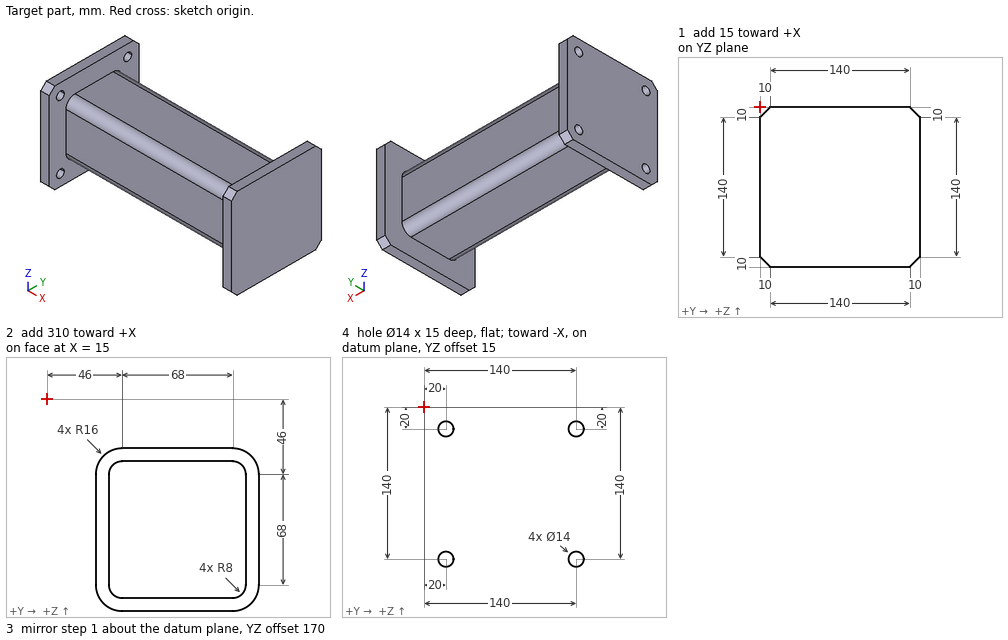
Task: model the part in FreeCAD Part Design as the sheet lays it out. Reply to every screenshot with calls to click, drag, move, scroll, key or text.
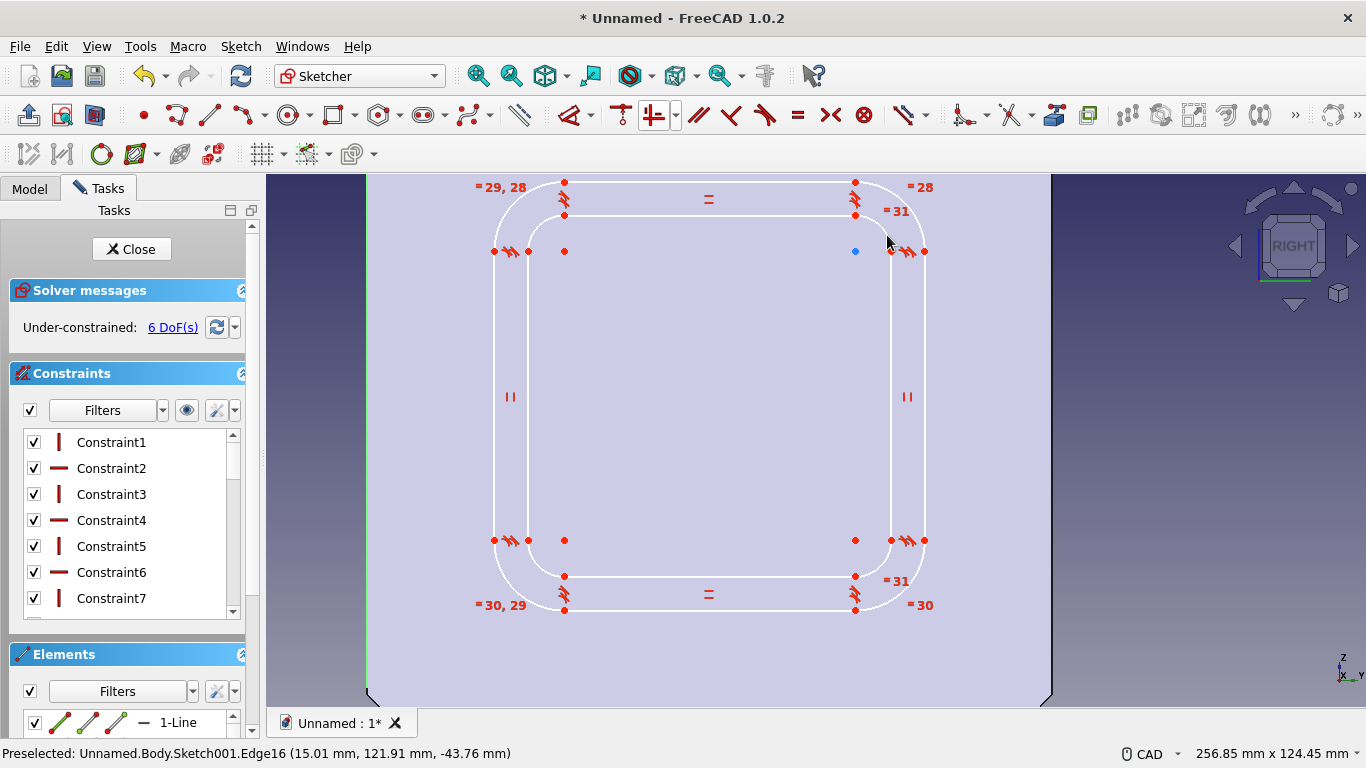
click(568, 116)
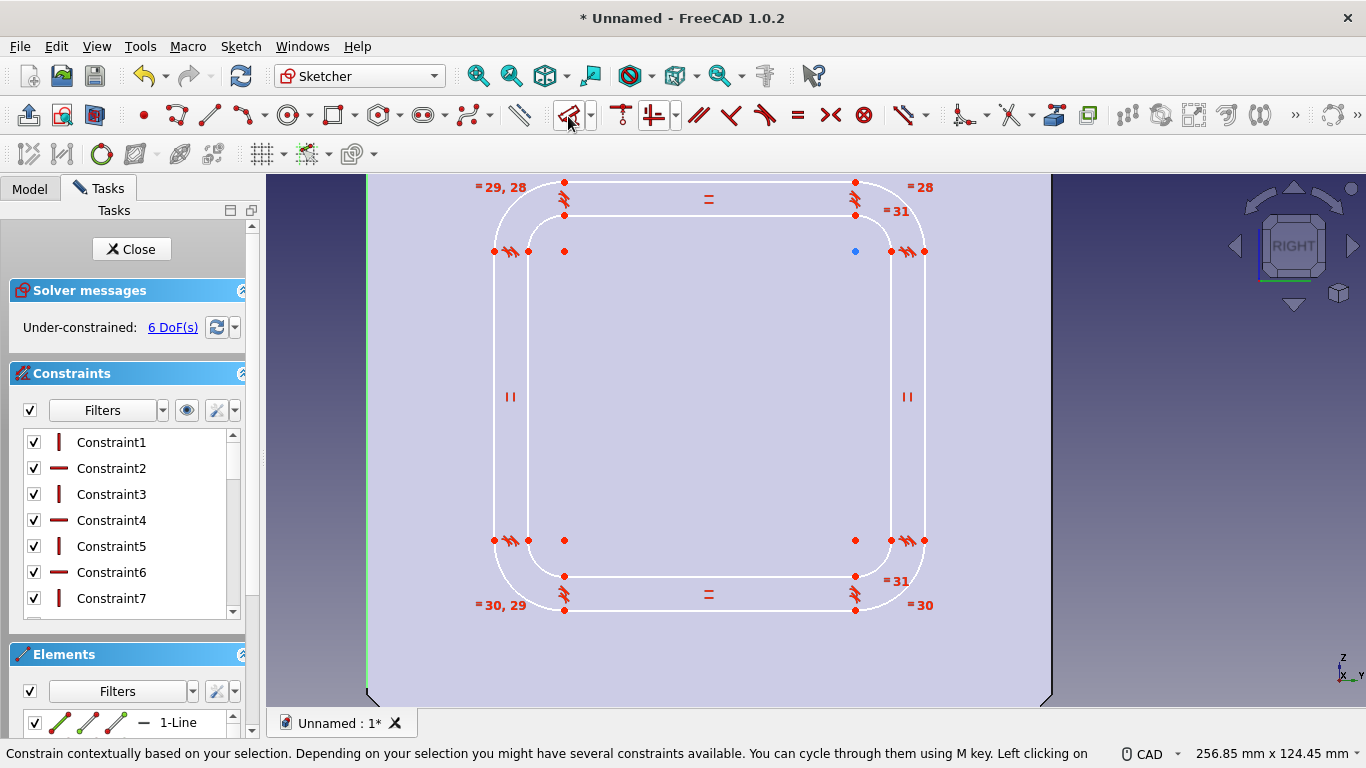
click(917, 220)
click(945, 205)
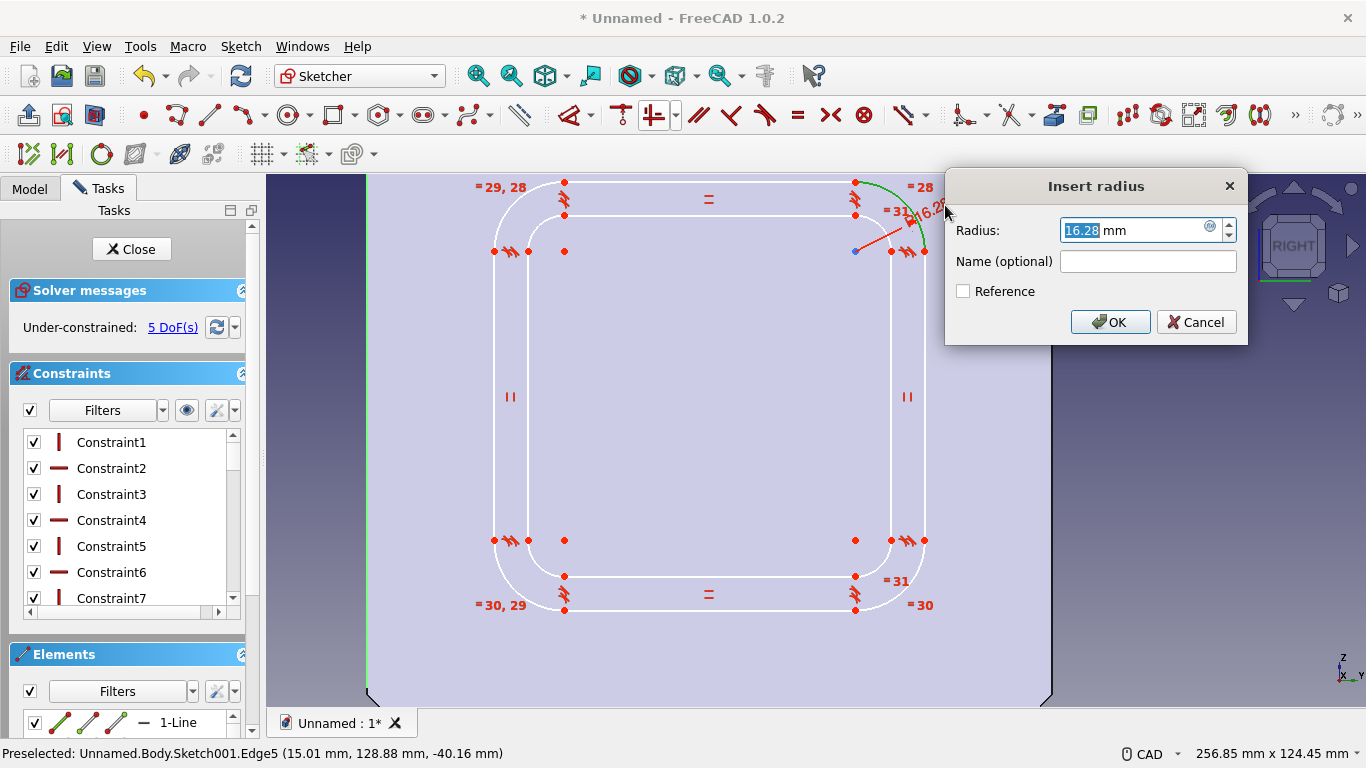
text(16)
key(Return)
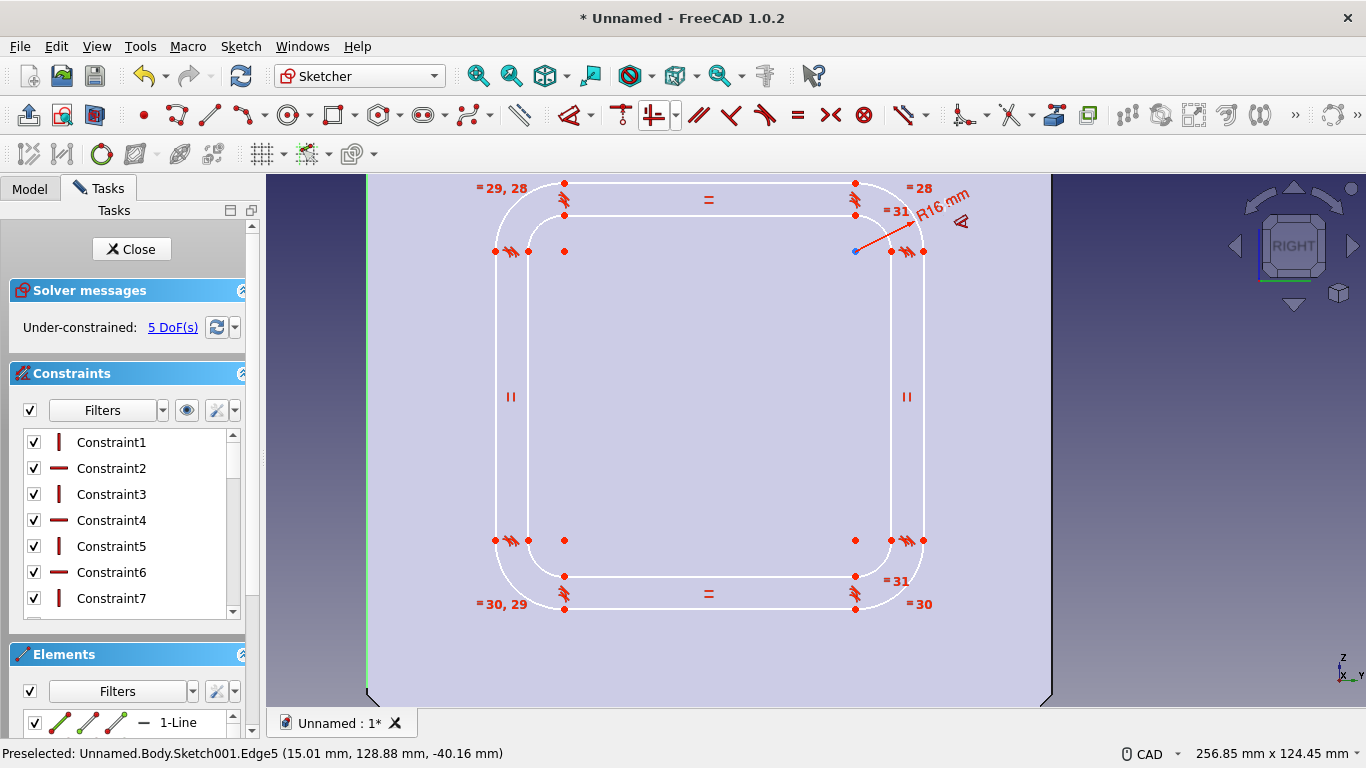
click(871, 573)
click(825, 480)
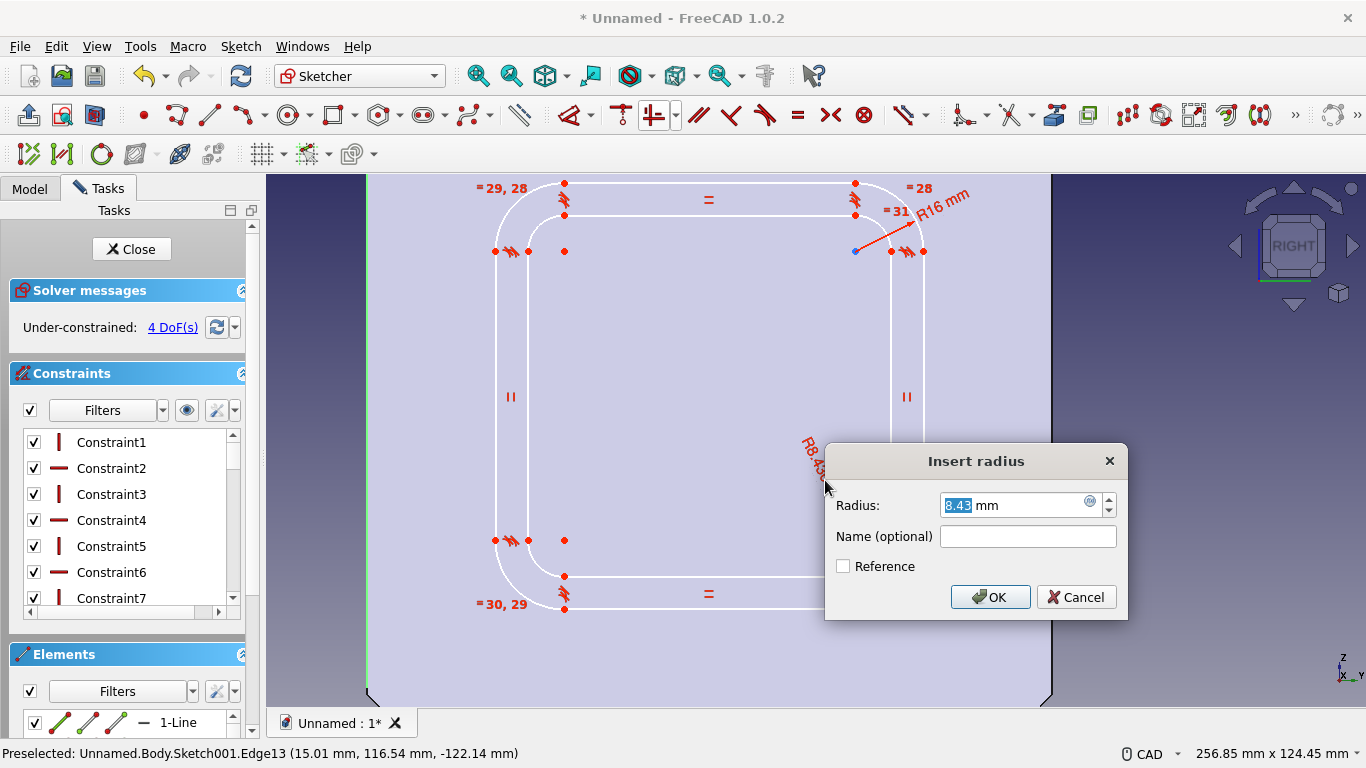
text(8)
key(Return)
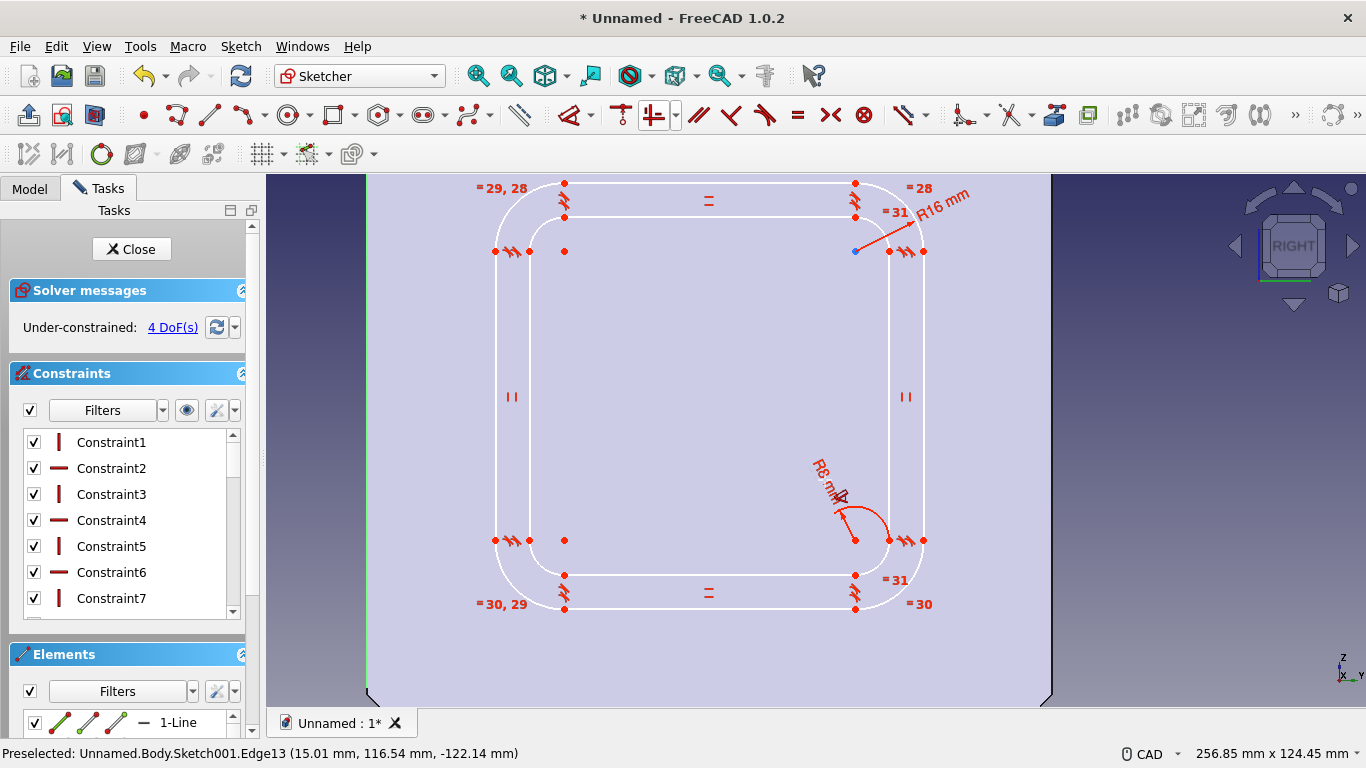
click(924, 454)
click(958, 396)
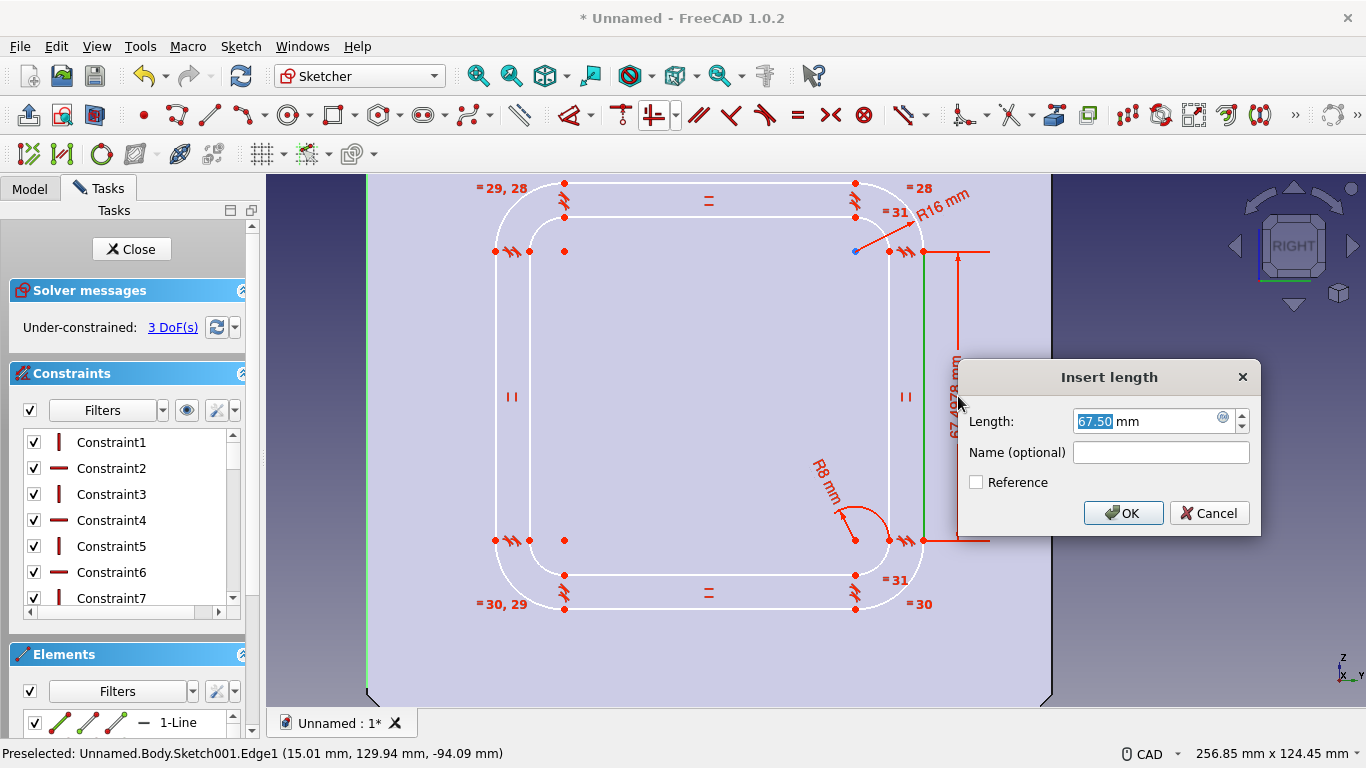
text(68)
key(Return)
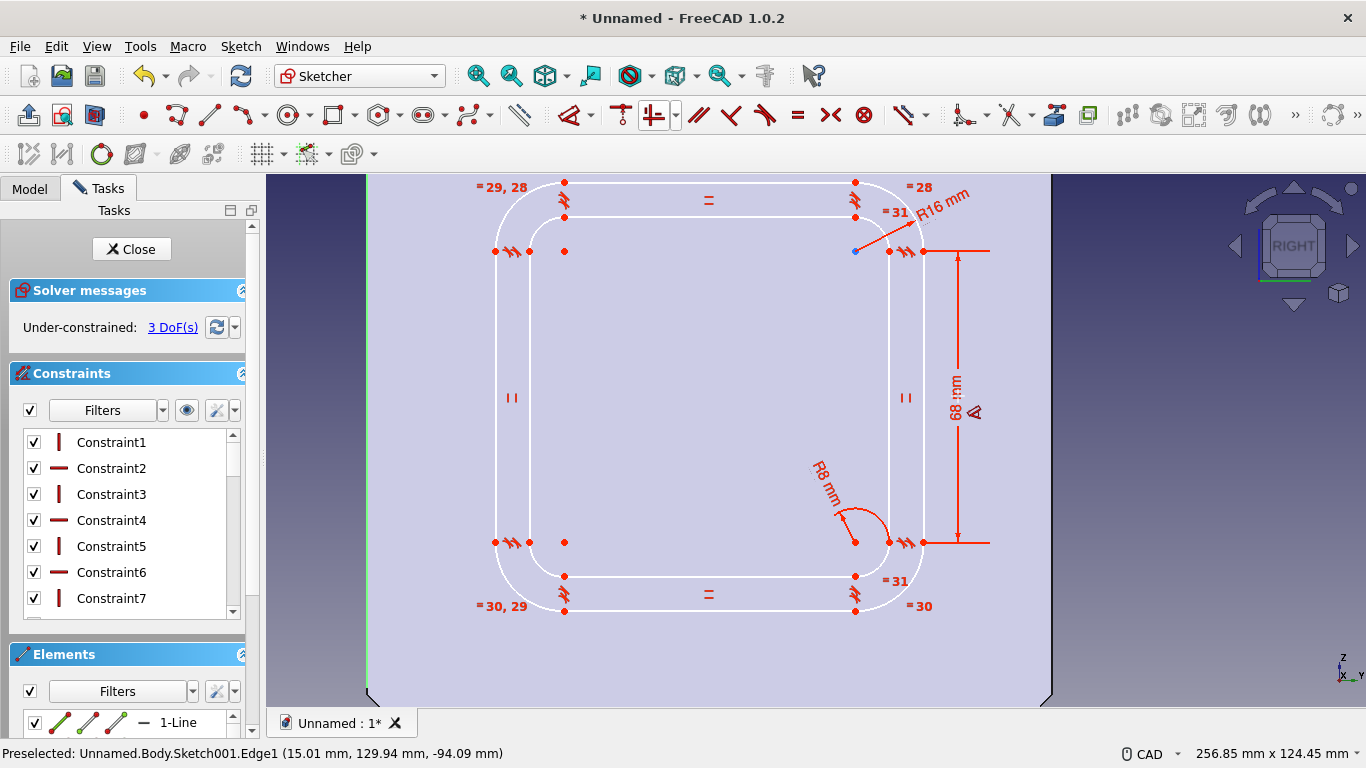
scroll(872, 574, down, 3)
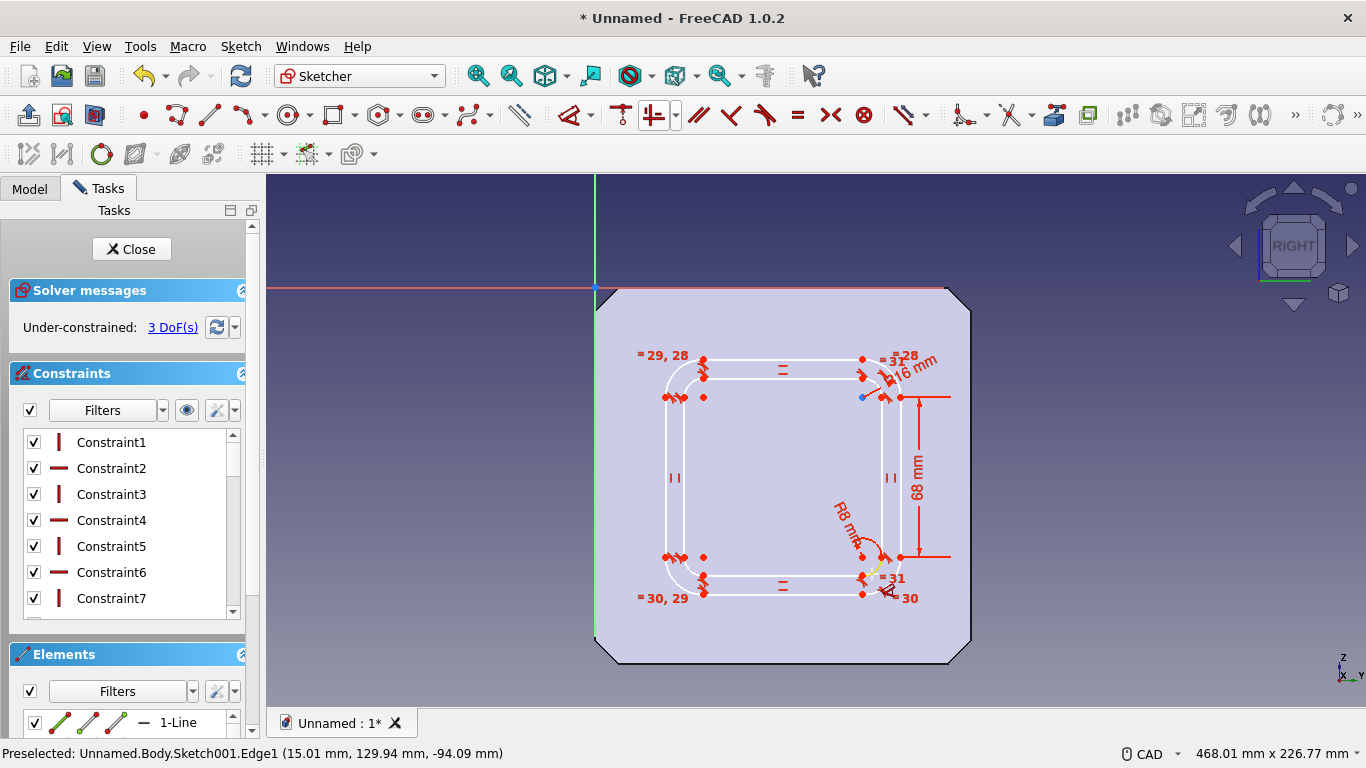
click(815, 360)
click(783, 326)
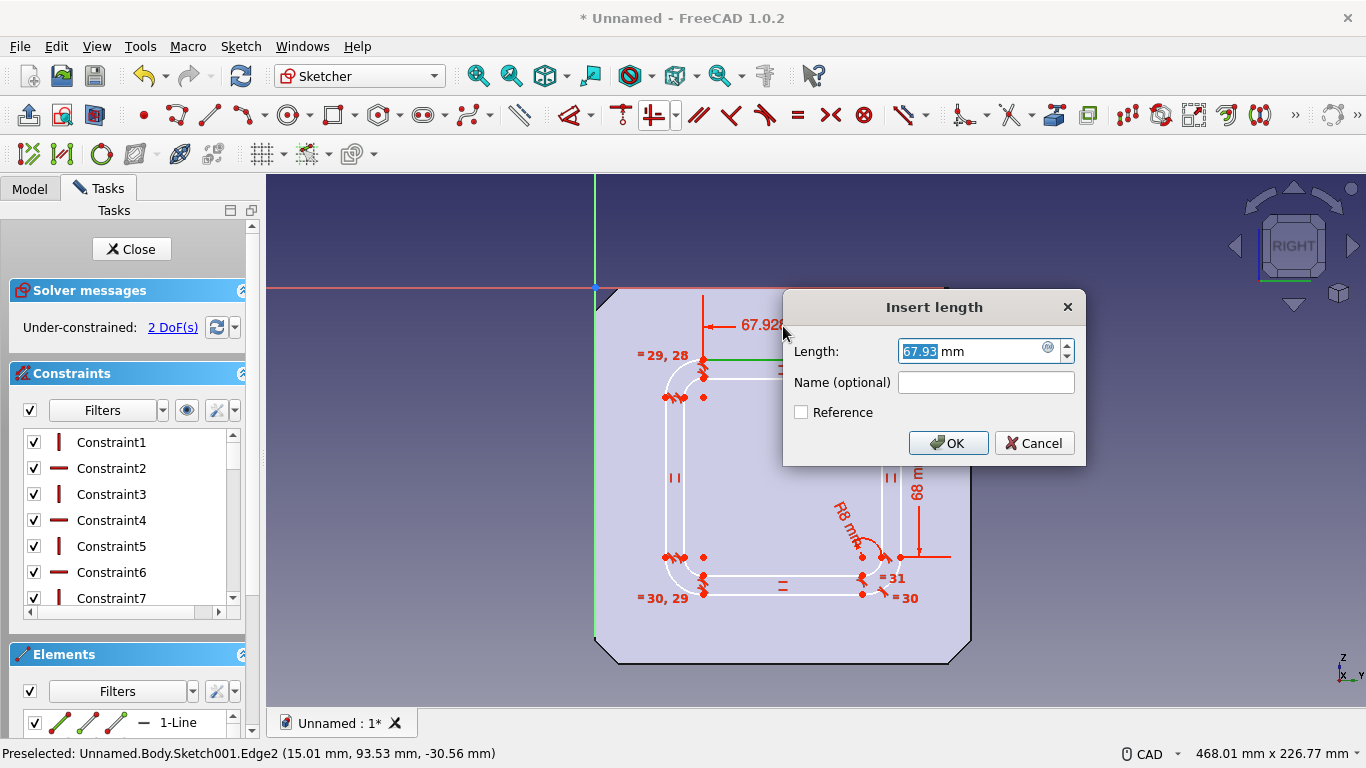
text(68)
key(Return)